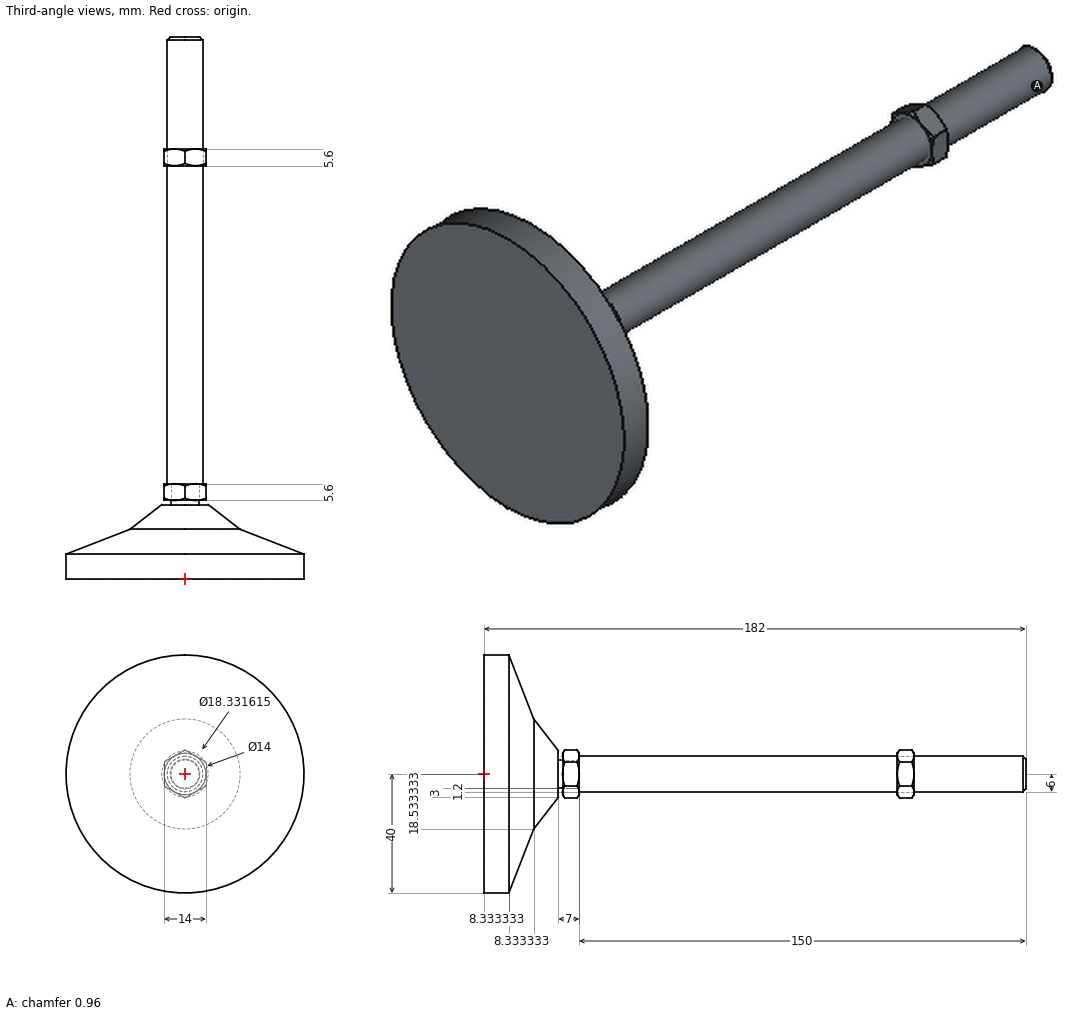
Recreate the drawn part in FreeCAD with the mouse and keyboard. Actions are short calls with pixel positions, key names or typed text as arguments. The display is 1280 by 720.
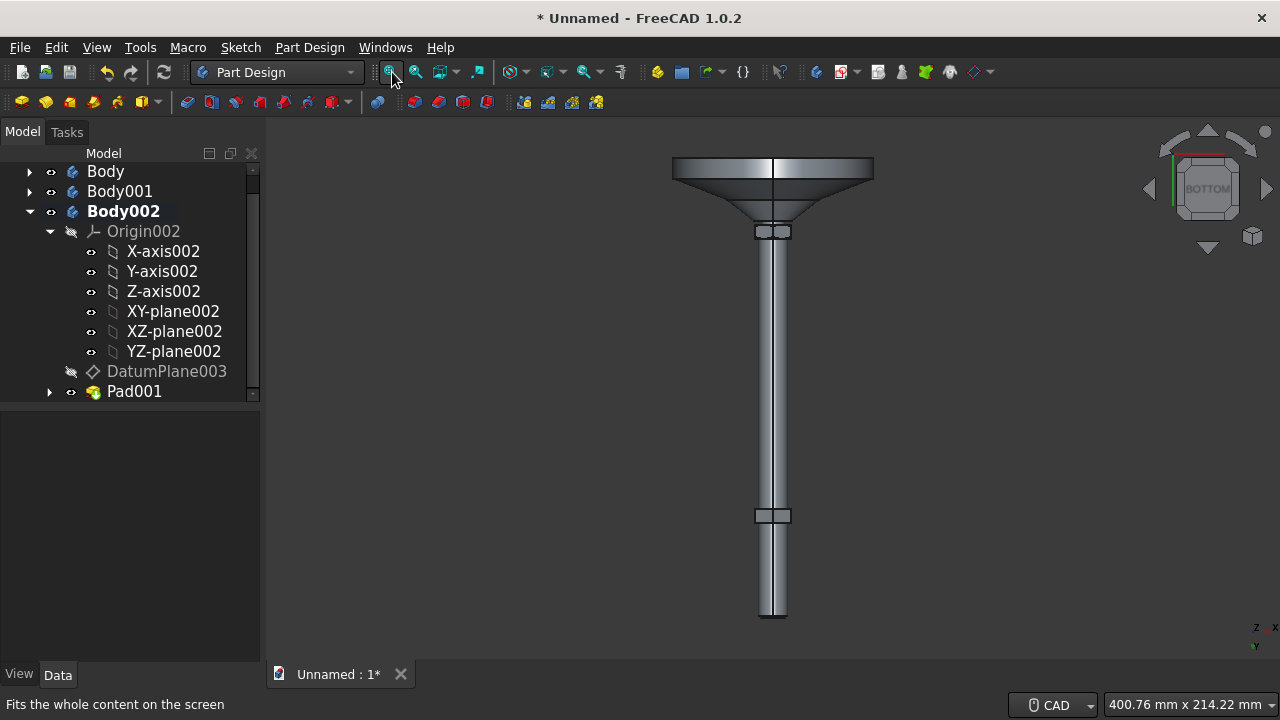
click(392, 72)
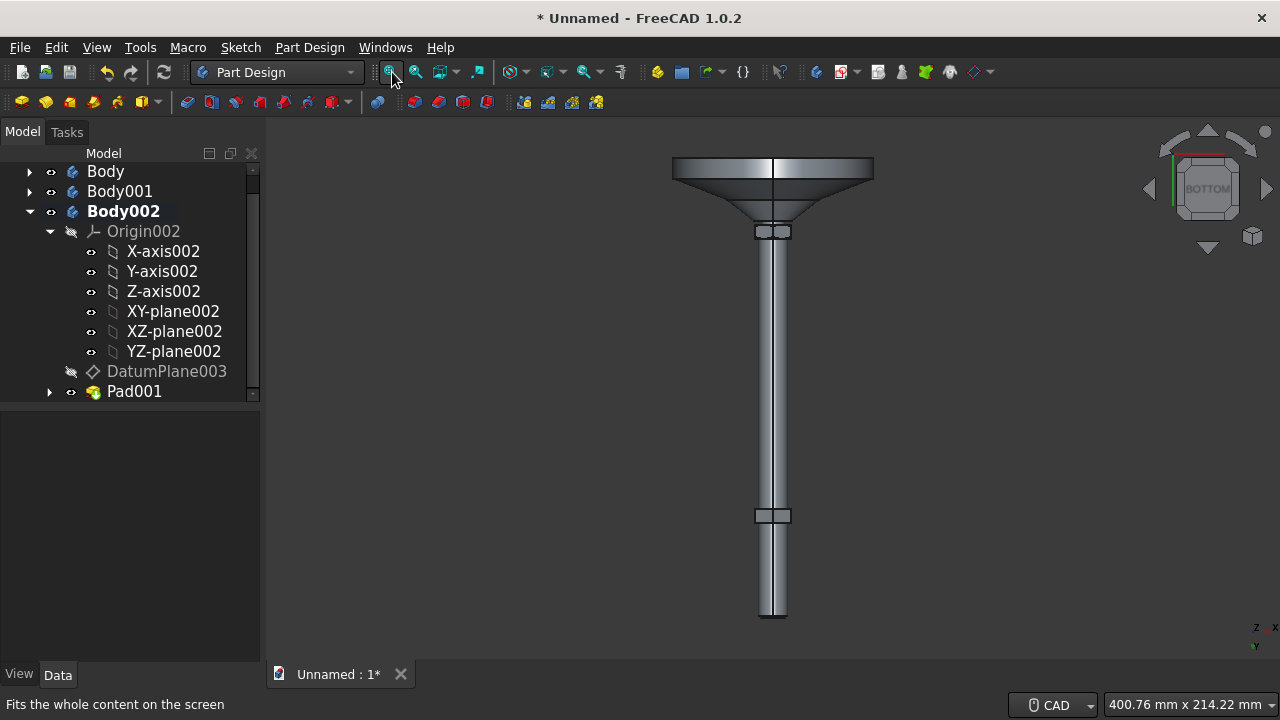
key(3)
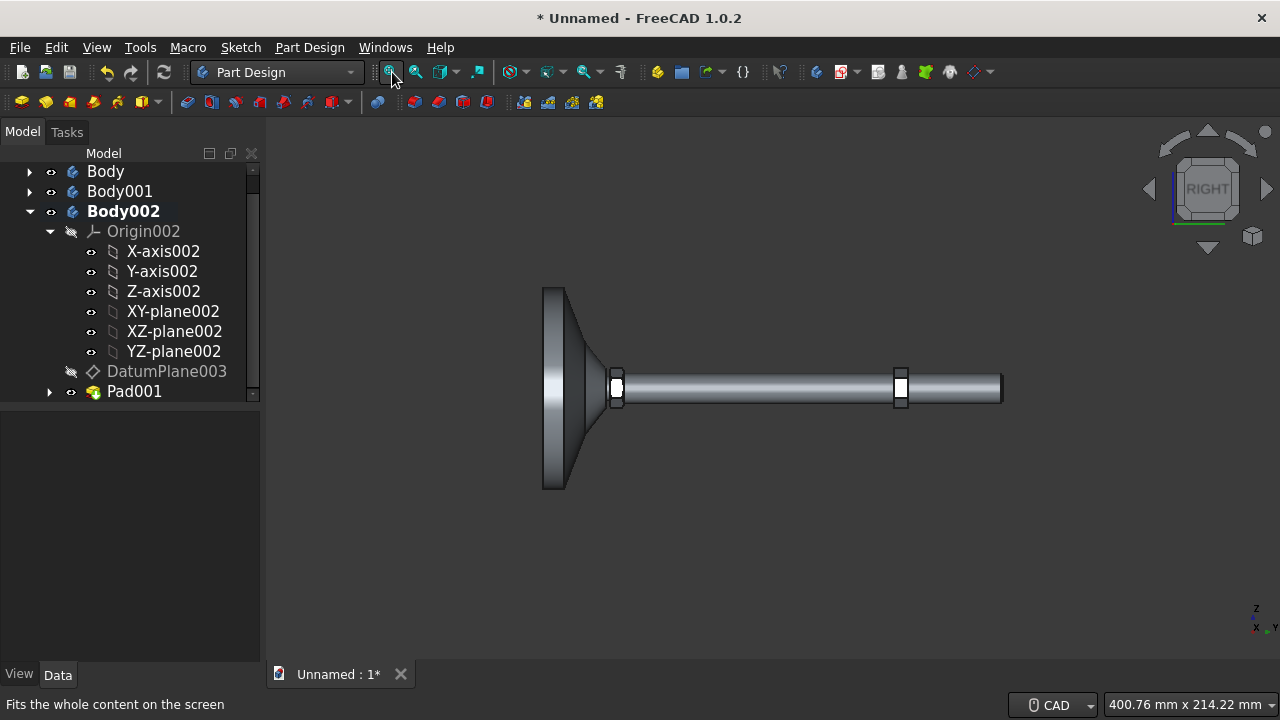
click(392, 72)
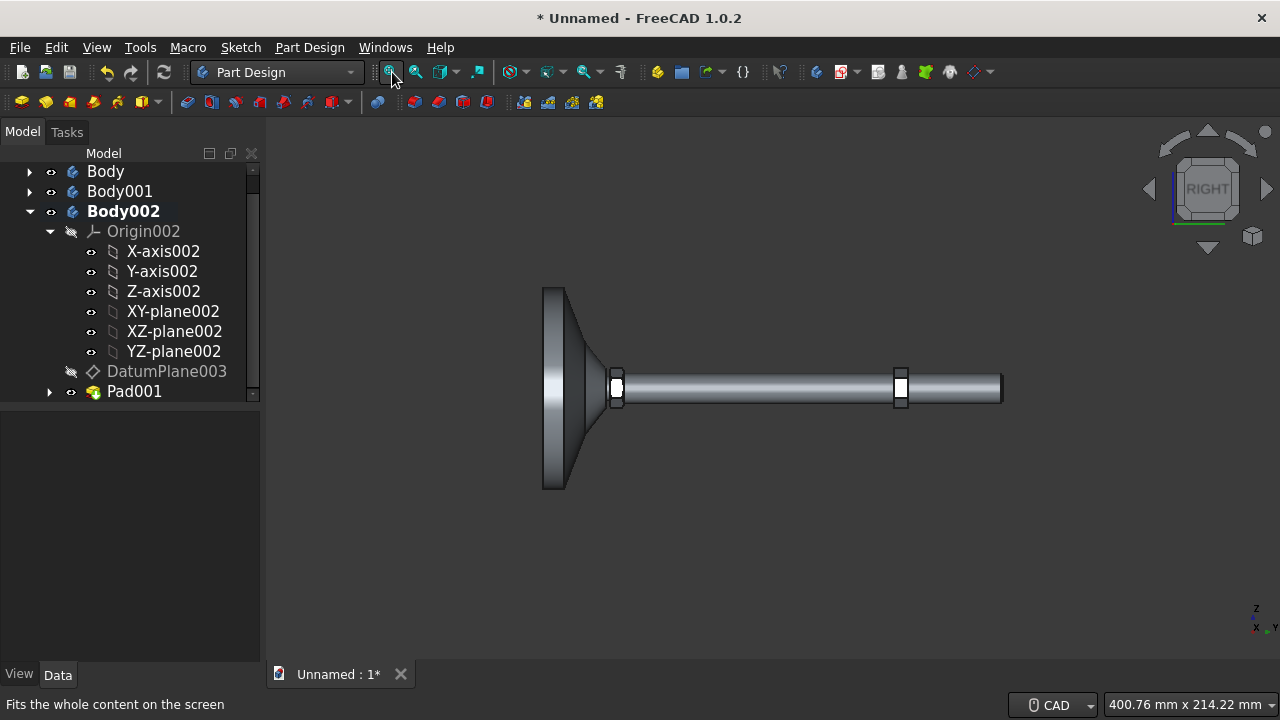
click(136, 332)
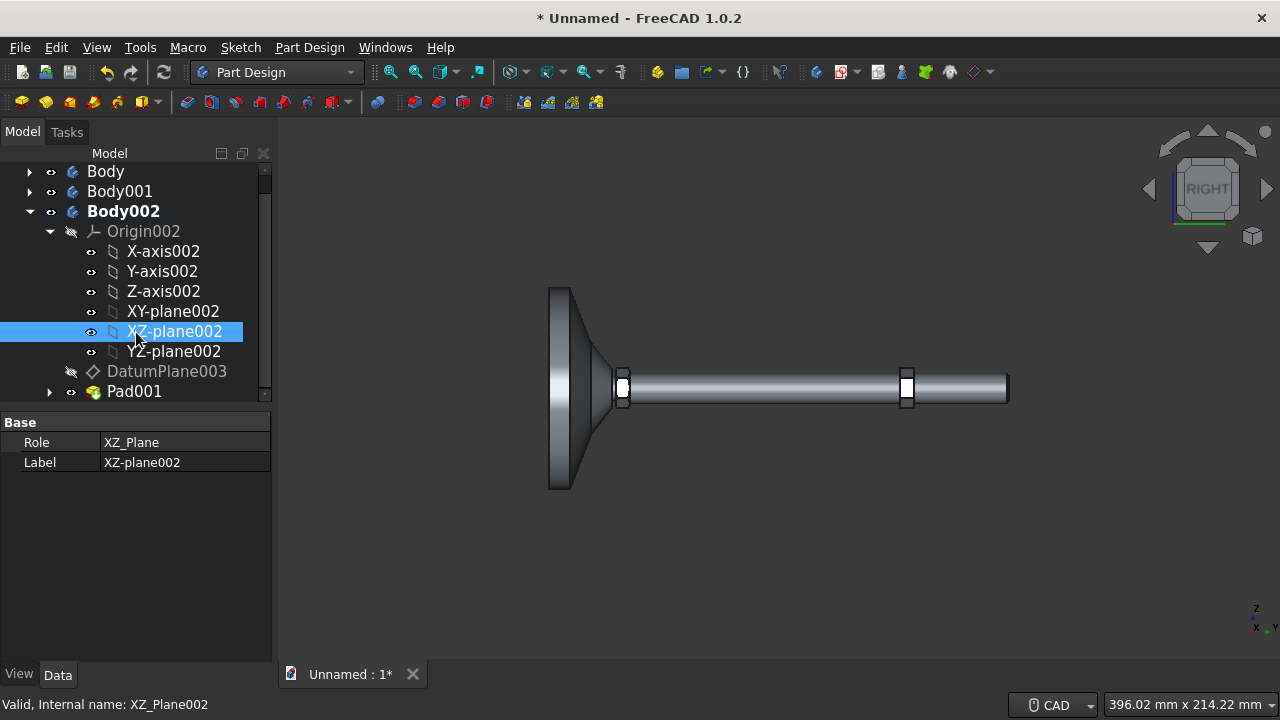
click(974, 72)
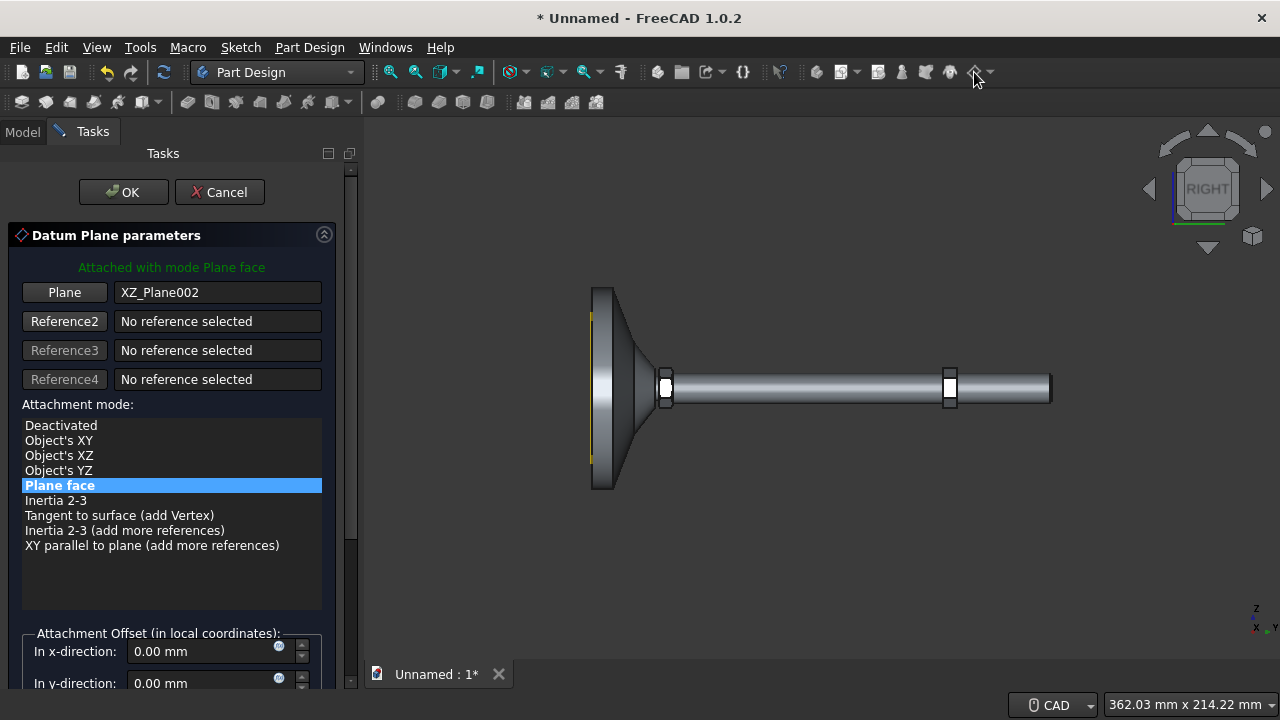
scroll(351, 426, down, 2)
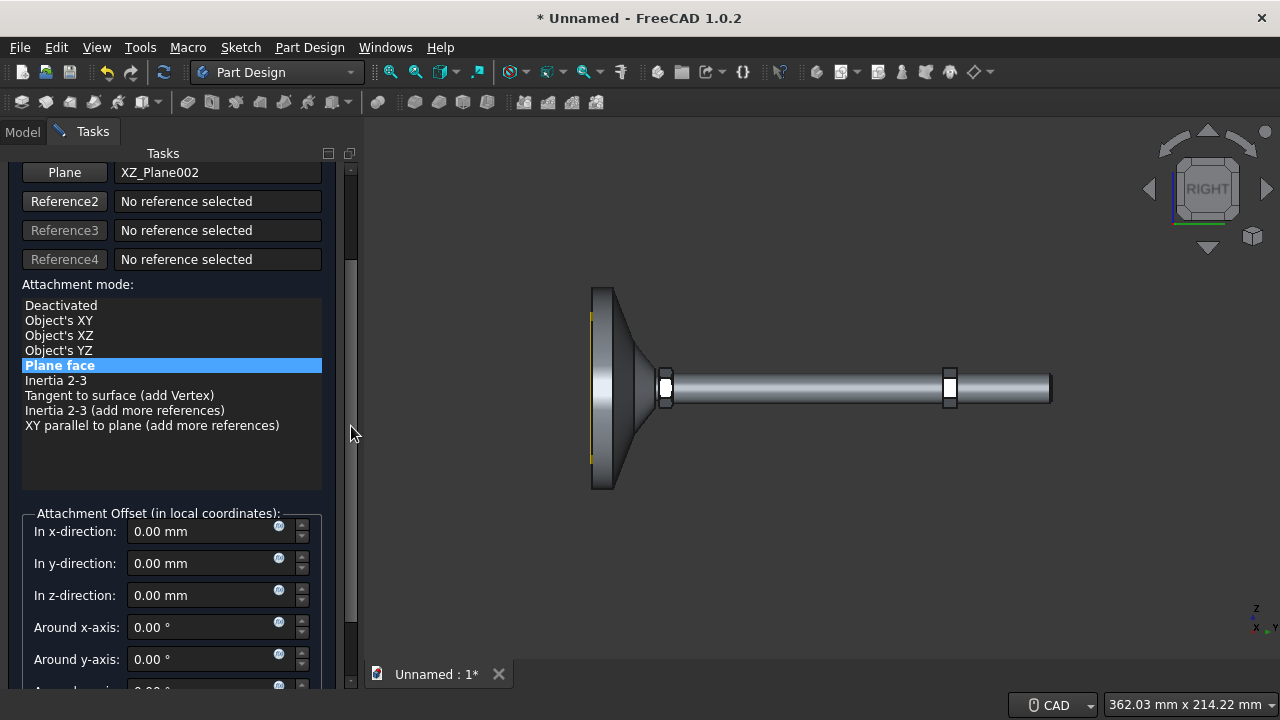
triple_click(210, 595)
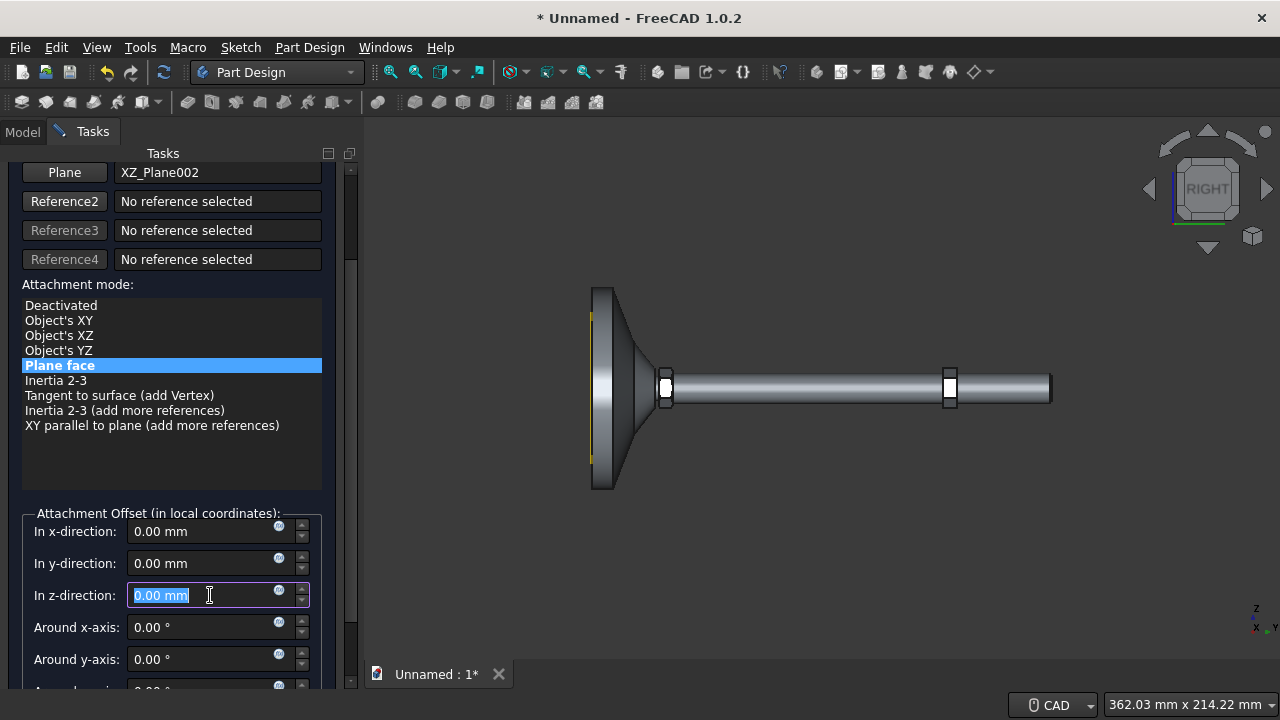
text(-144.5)
key(Tab)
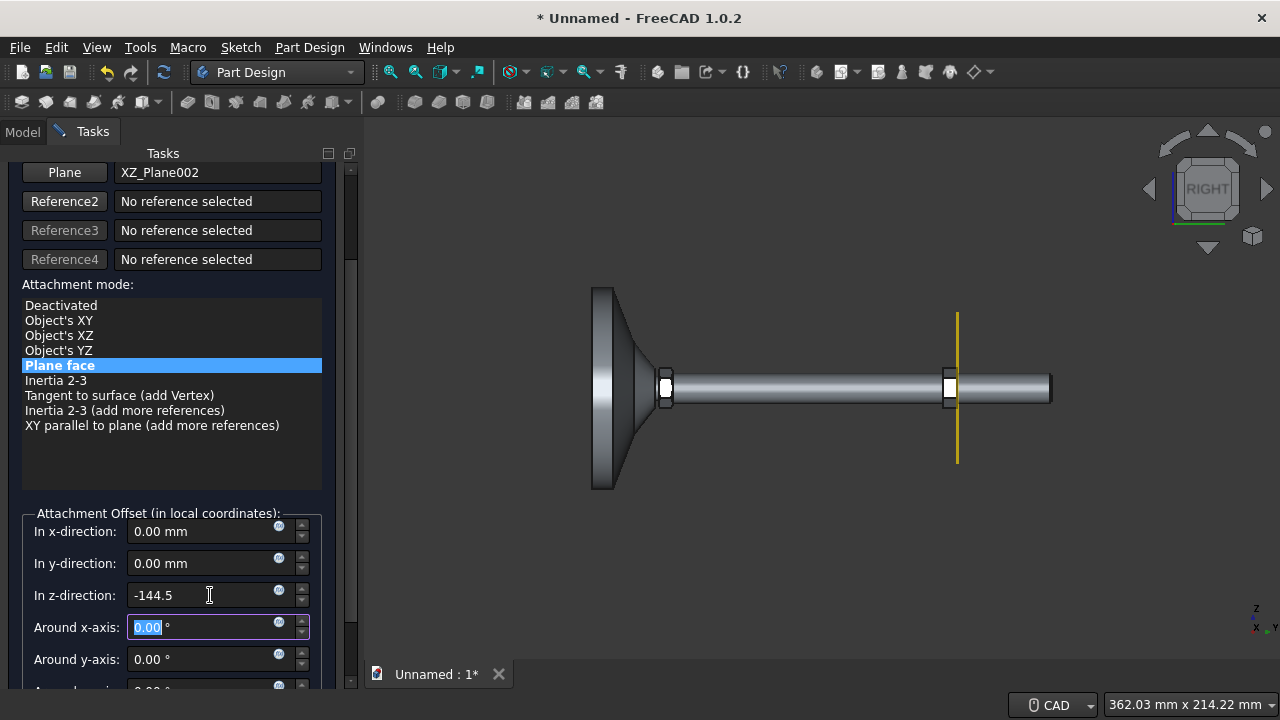
scroll(351, 426, up, 3)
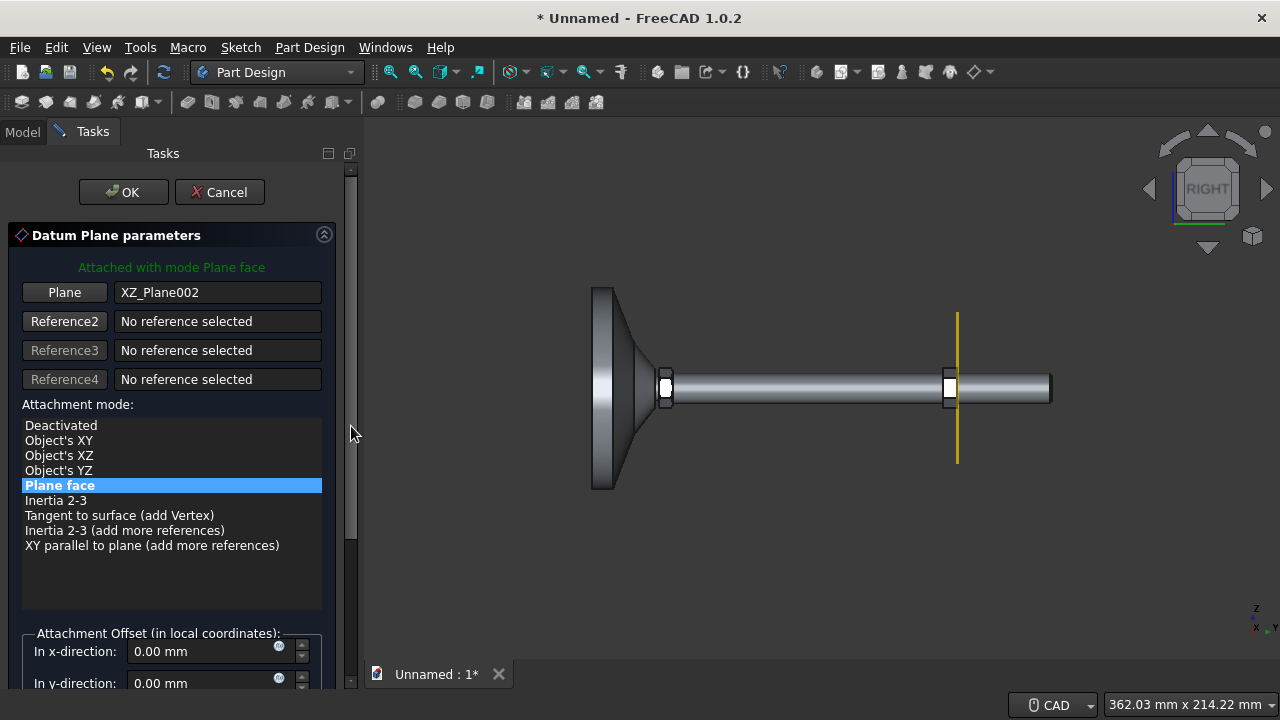
click(124, 192)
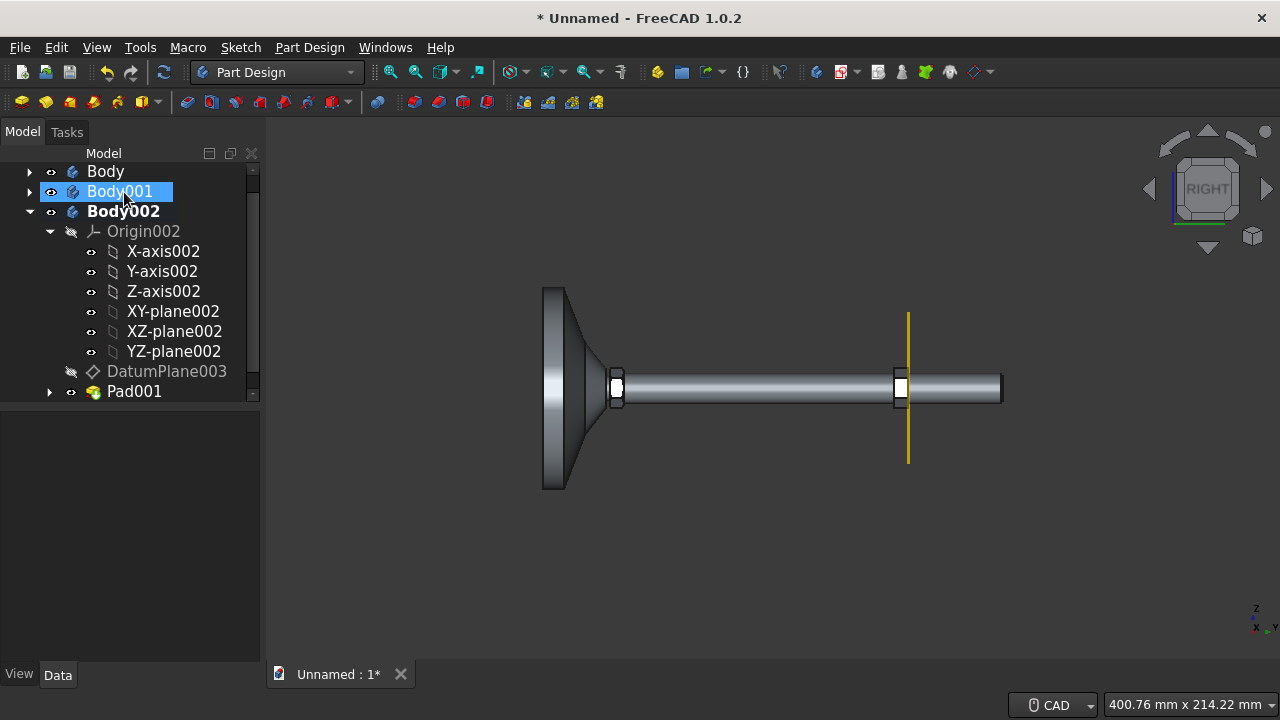
scroll(120, 287, down, 3)